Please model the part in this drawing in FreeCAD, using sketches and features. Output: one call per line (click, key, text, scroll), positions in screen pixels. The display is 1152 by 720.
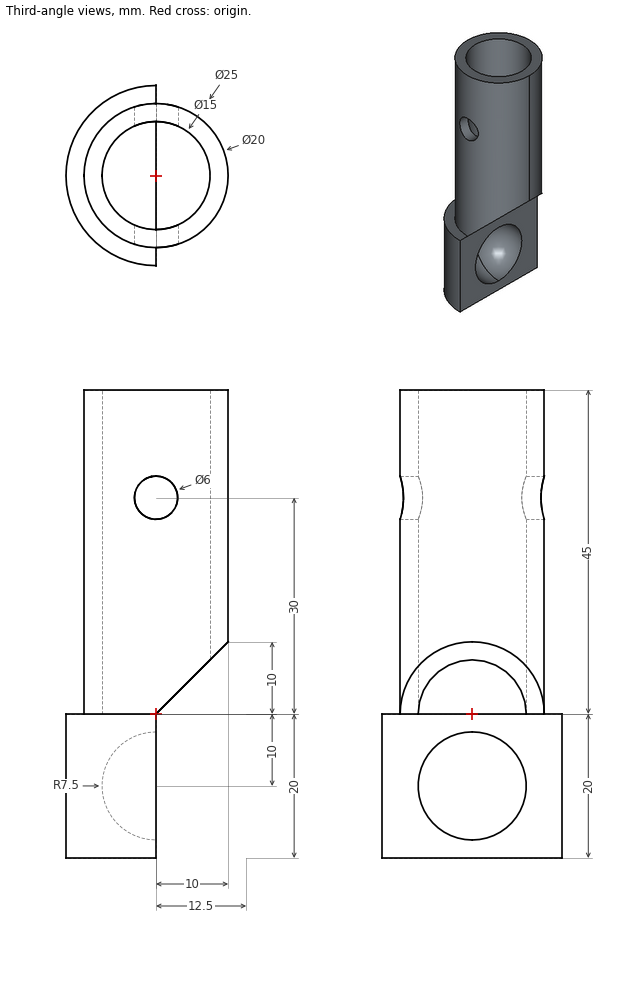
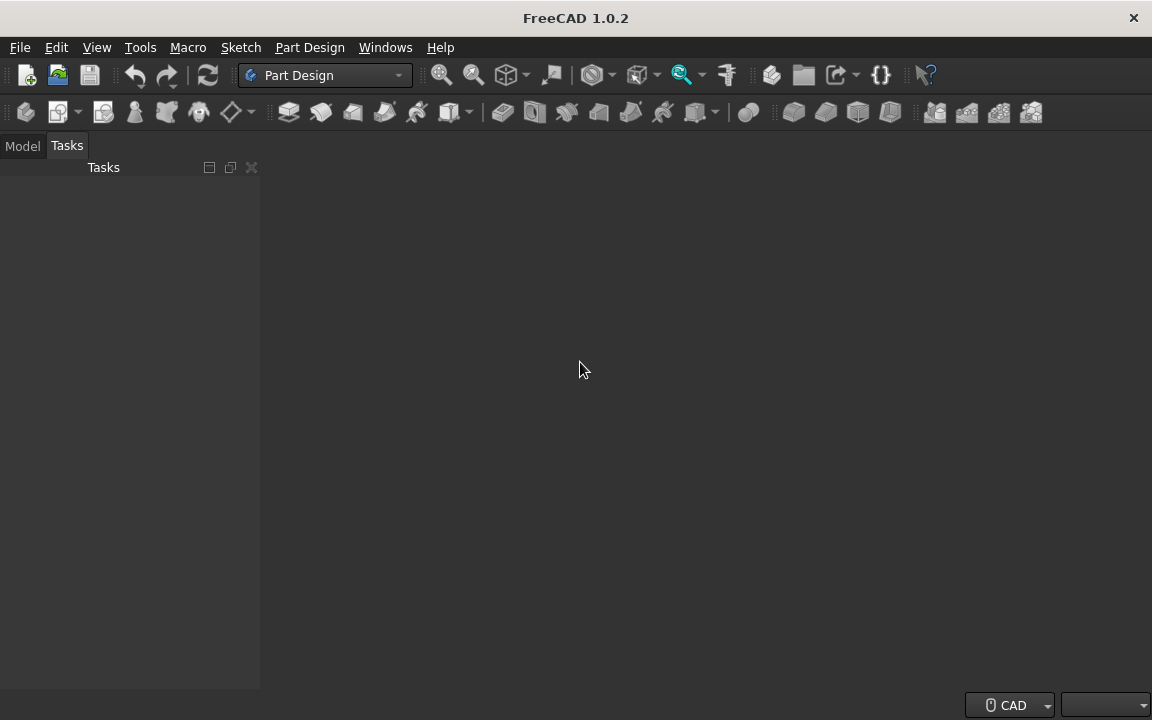
click(26, 76)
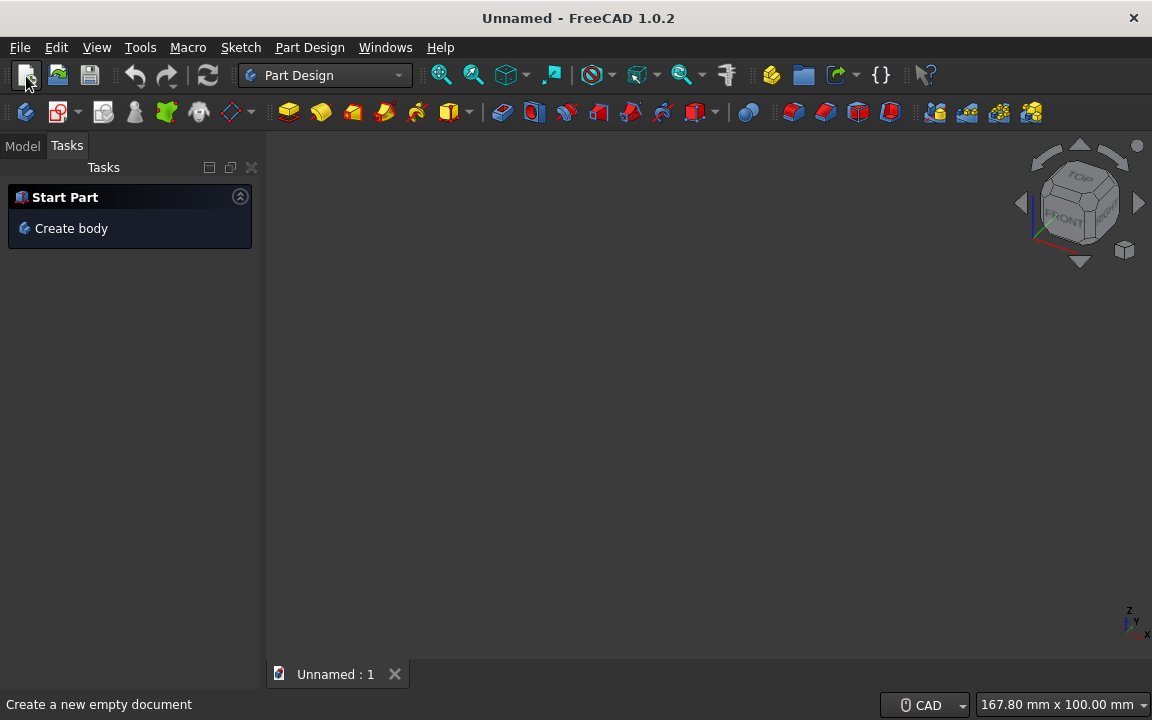
click(58, 112)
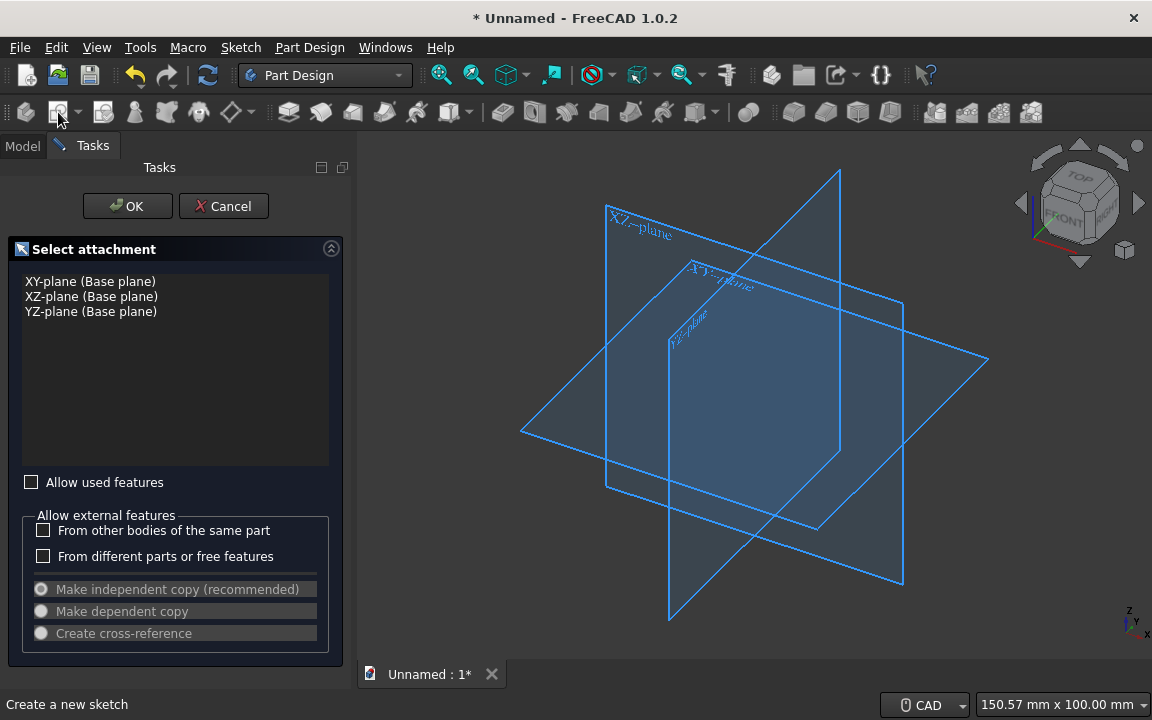
click(82, 282)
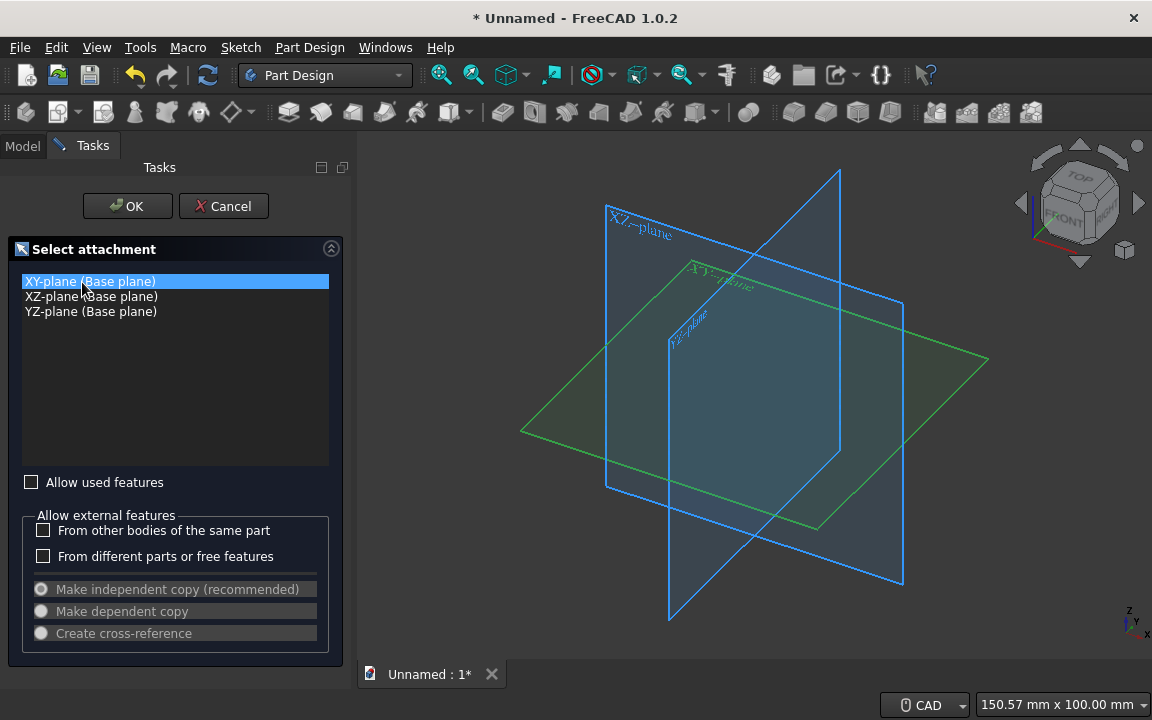
click(128, 206)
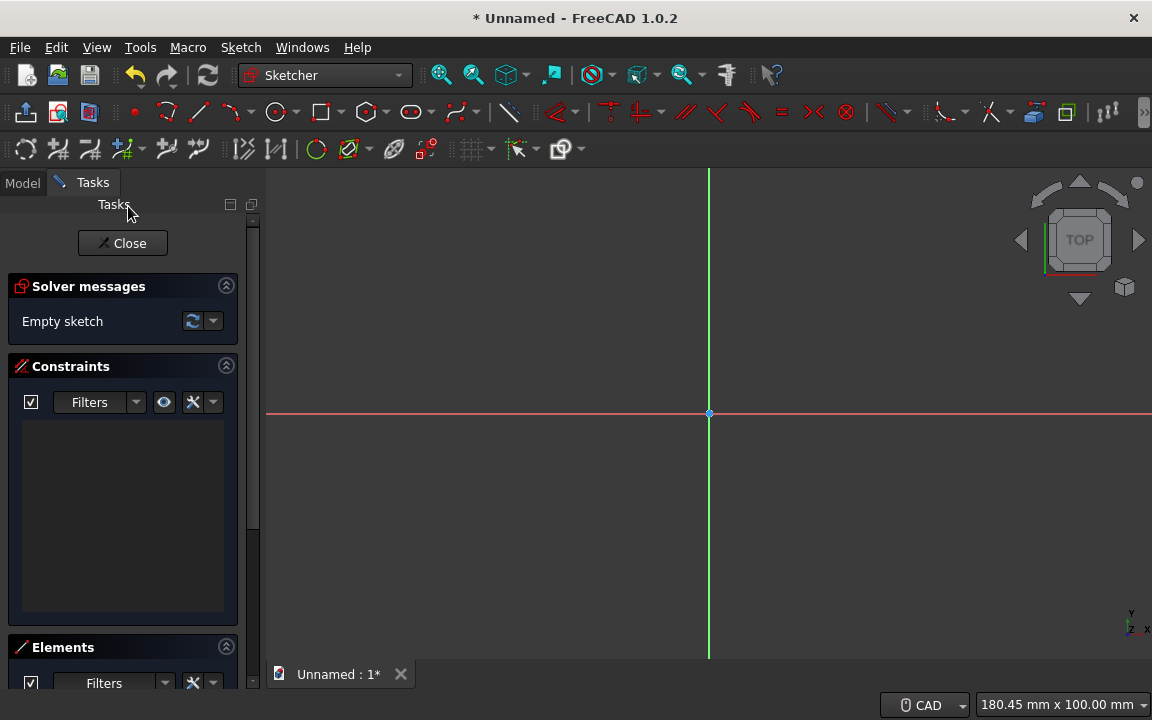
scroll(739, 414, up, 6)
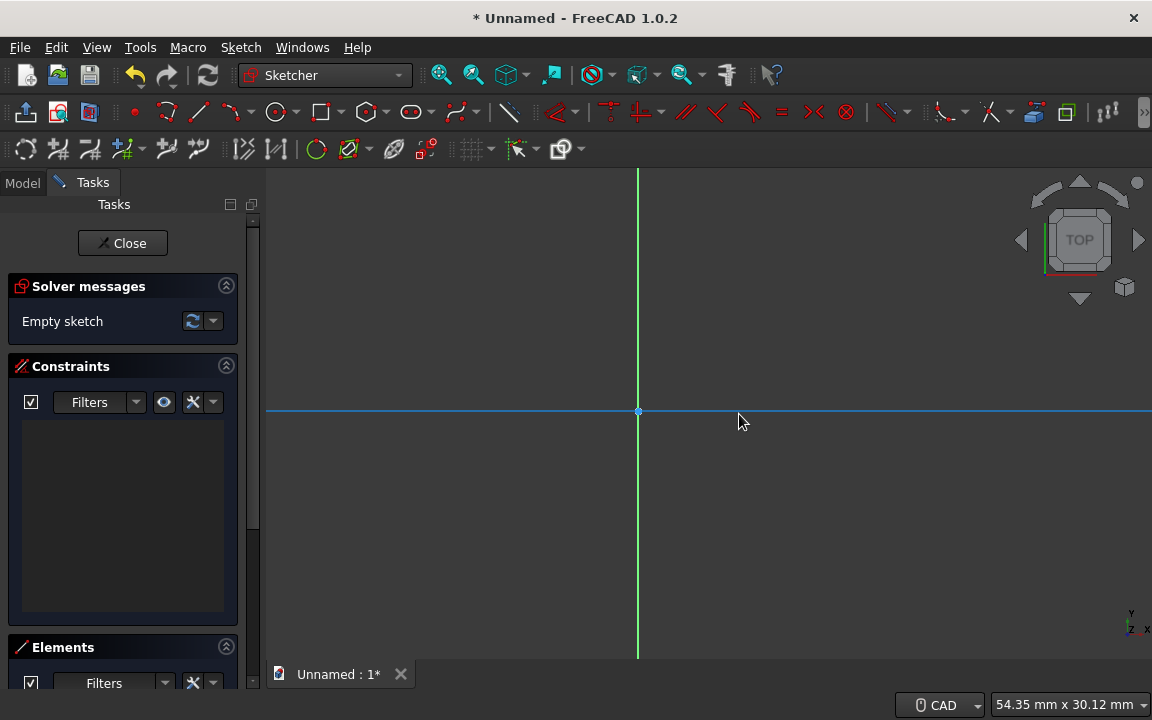
click(276, 112)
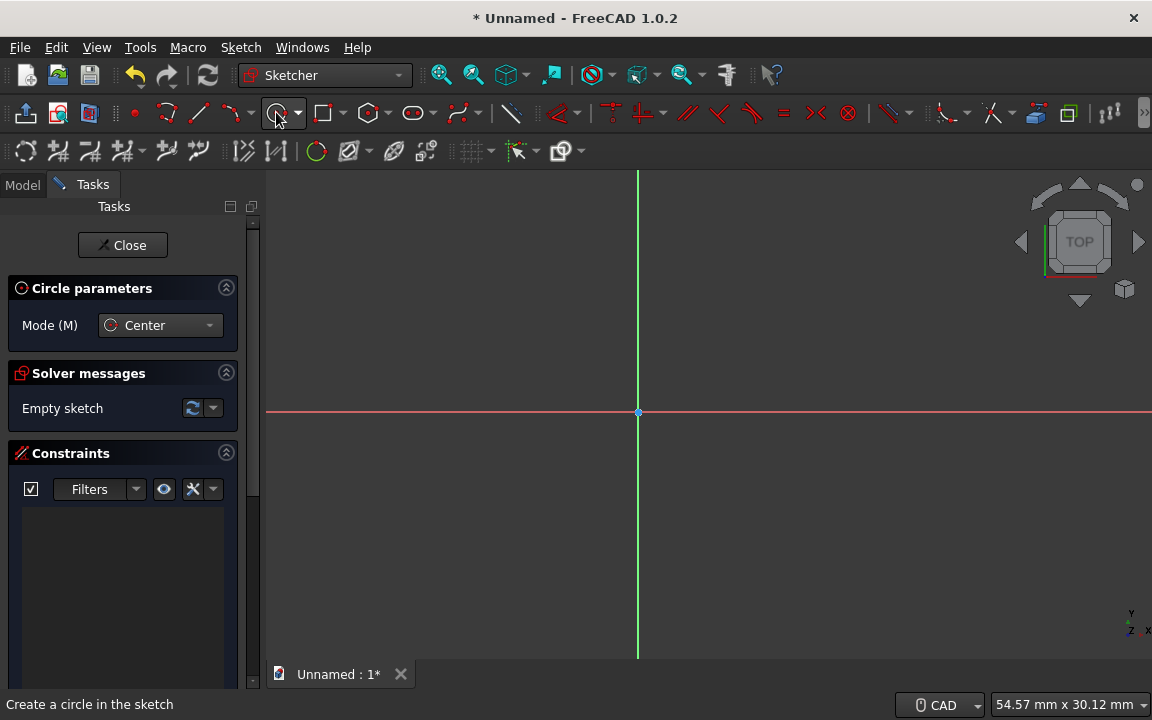
click(638, 412)
click(753, 297)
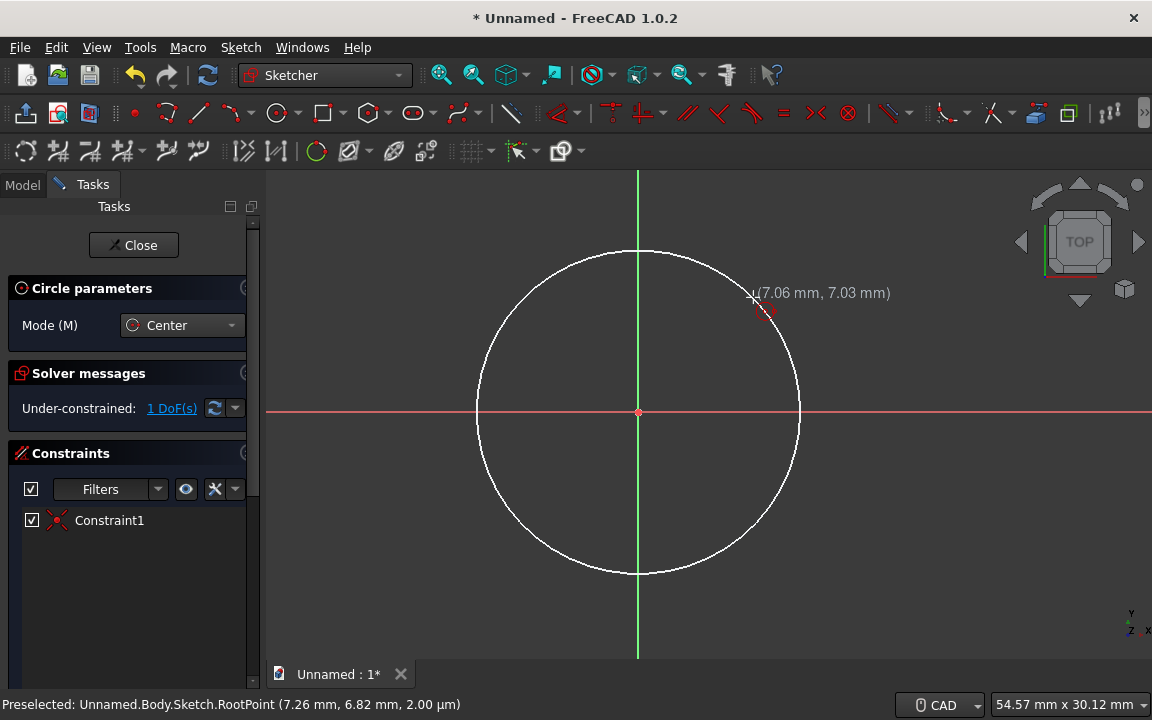
click(638, 412)
click(725, 326)
key(Escape)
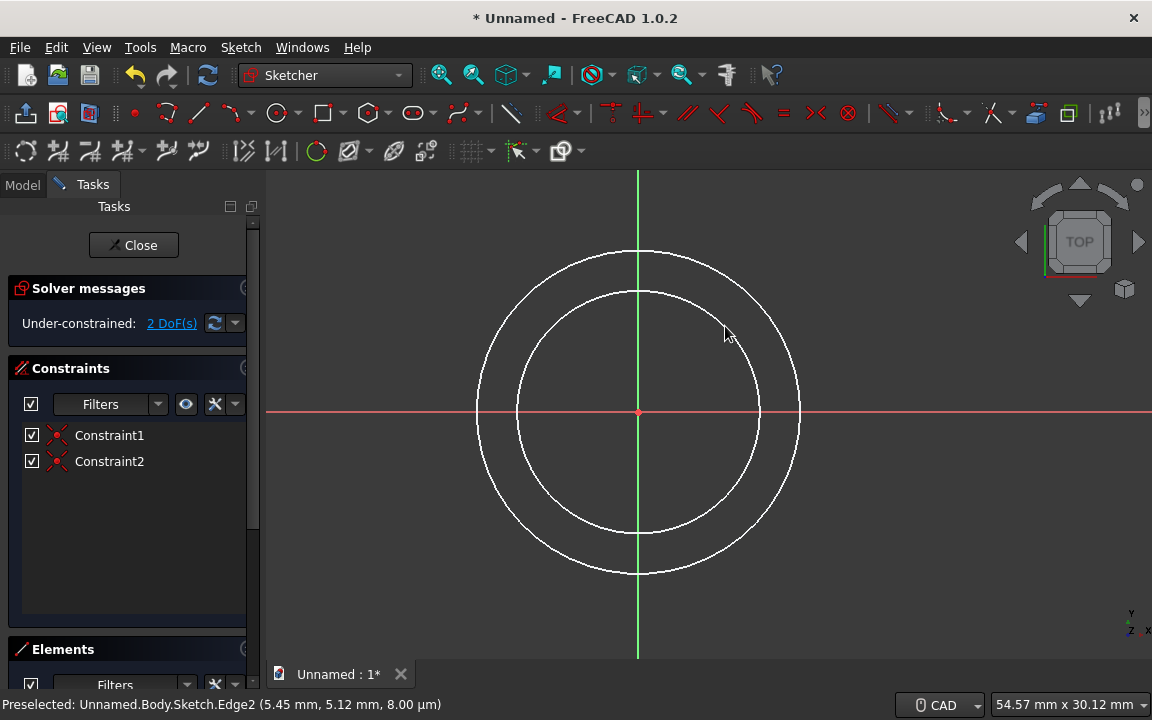
click(558, 114)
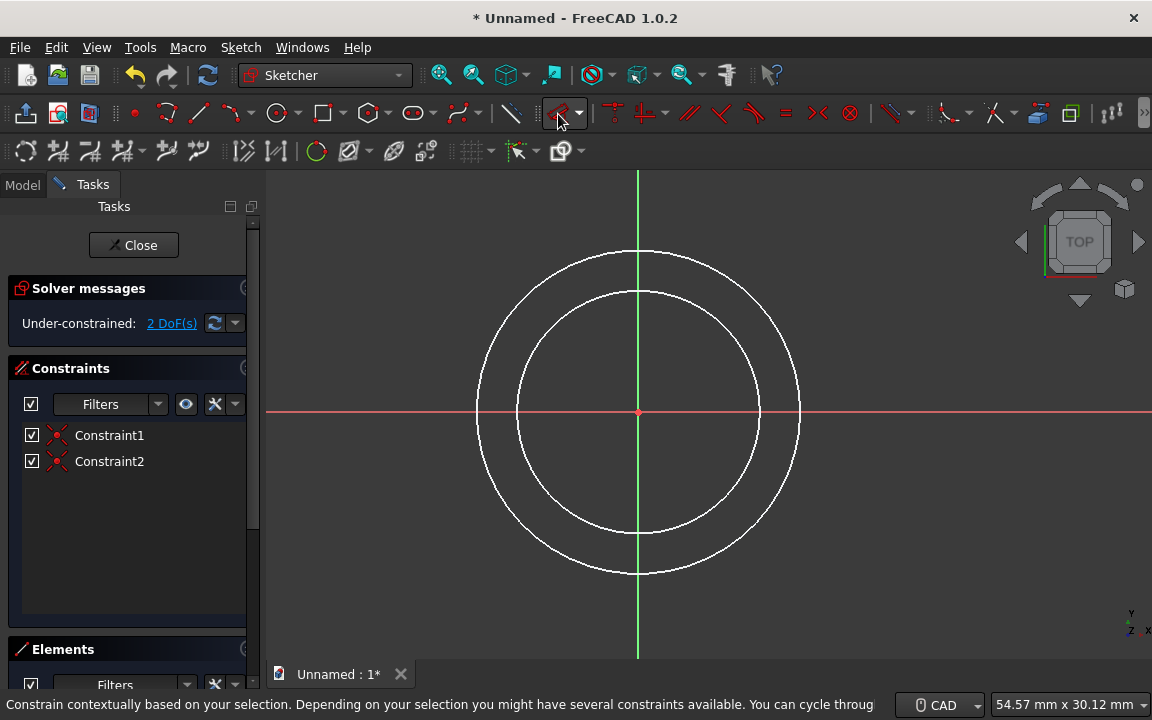
click(752, 297)
click(774, 274)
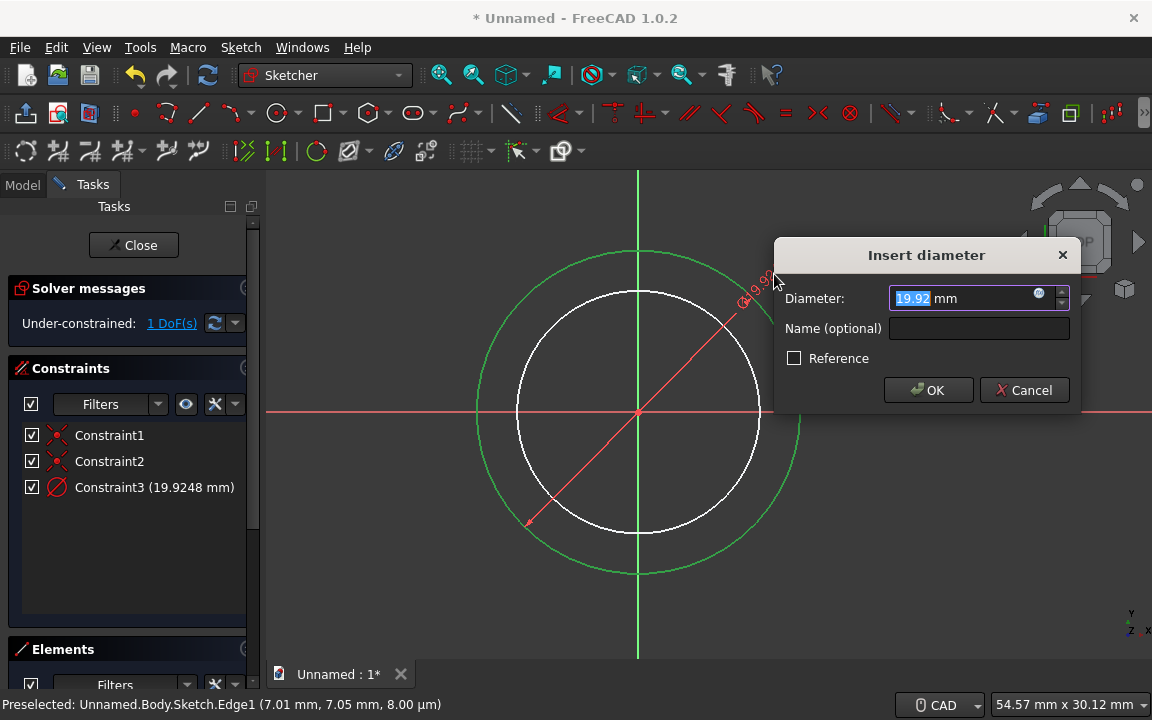
text(20)
key(Return)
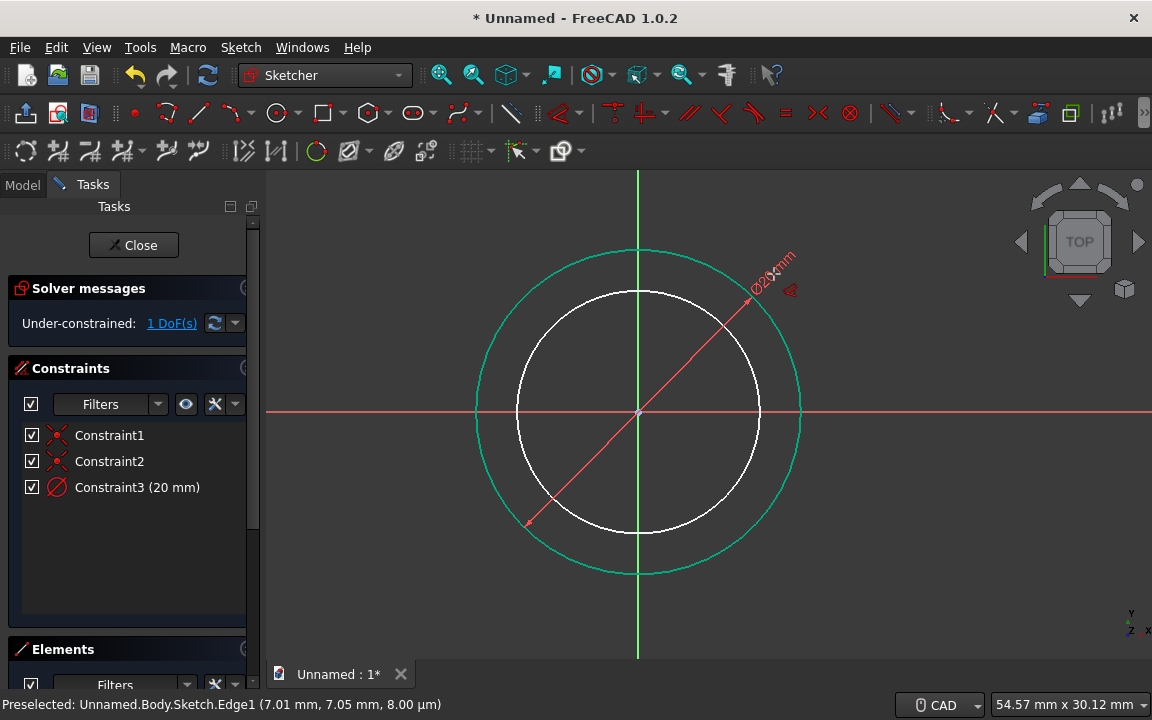
click(724, 326)
click(808, 362)